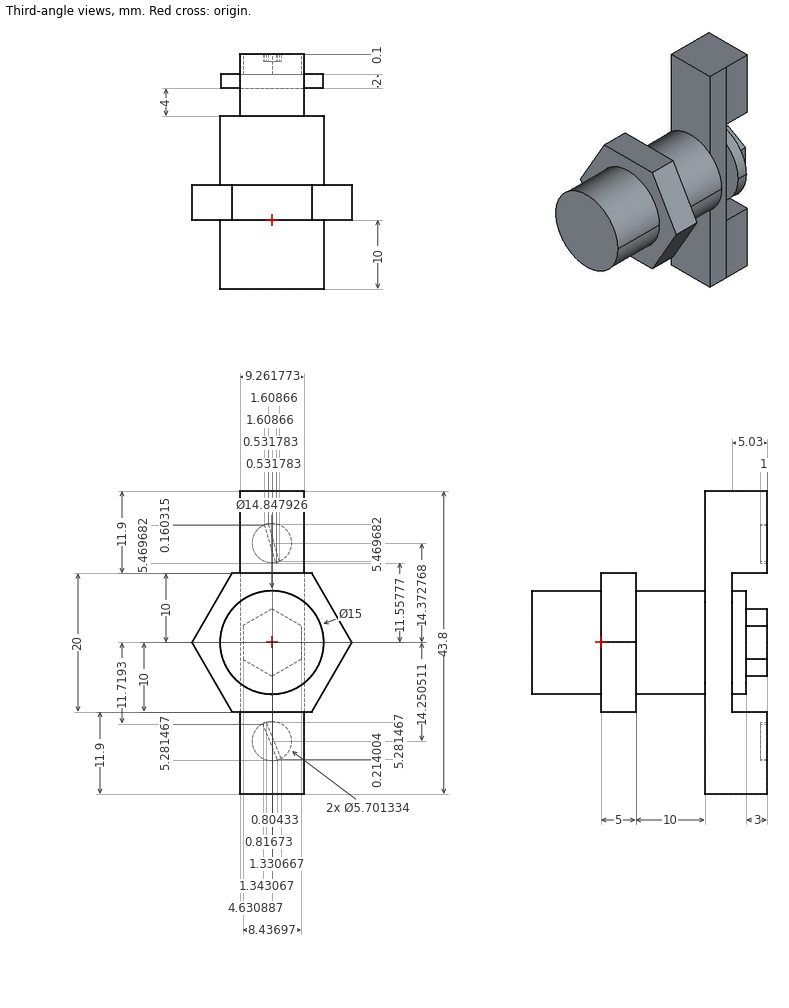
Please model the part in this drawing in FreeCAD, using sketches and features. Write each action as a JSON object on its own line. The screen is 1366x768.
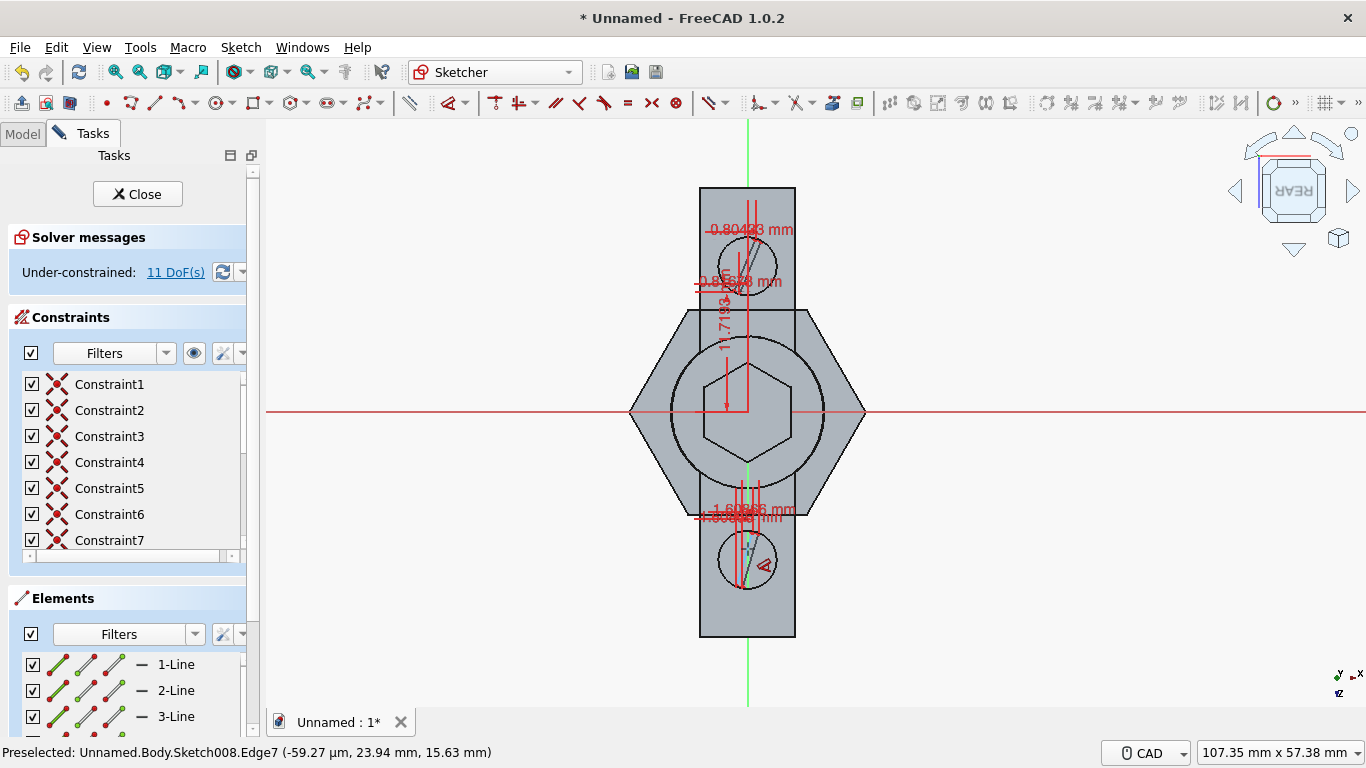
{"action": "scroll", "coordinate": [761, 241], "scroll_direction": "up", "scroll_amount": 6}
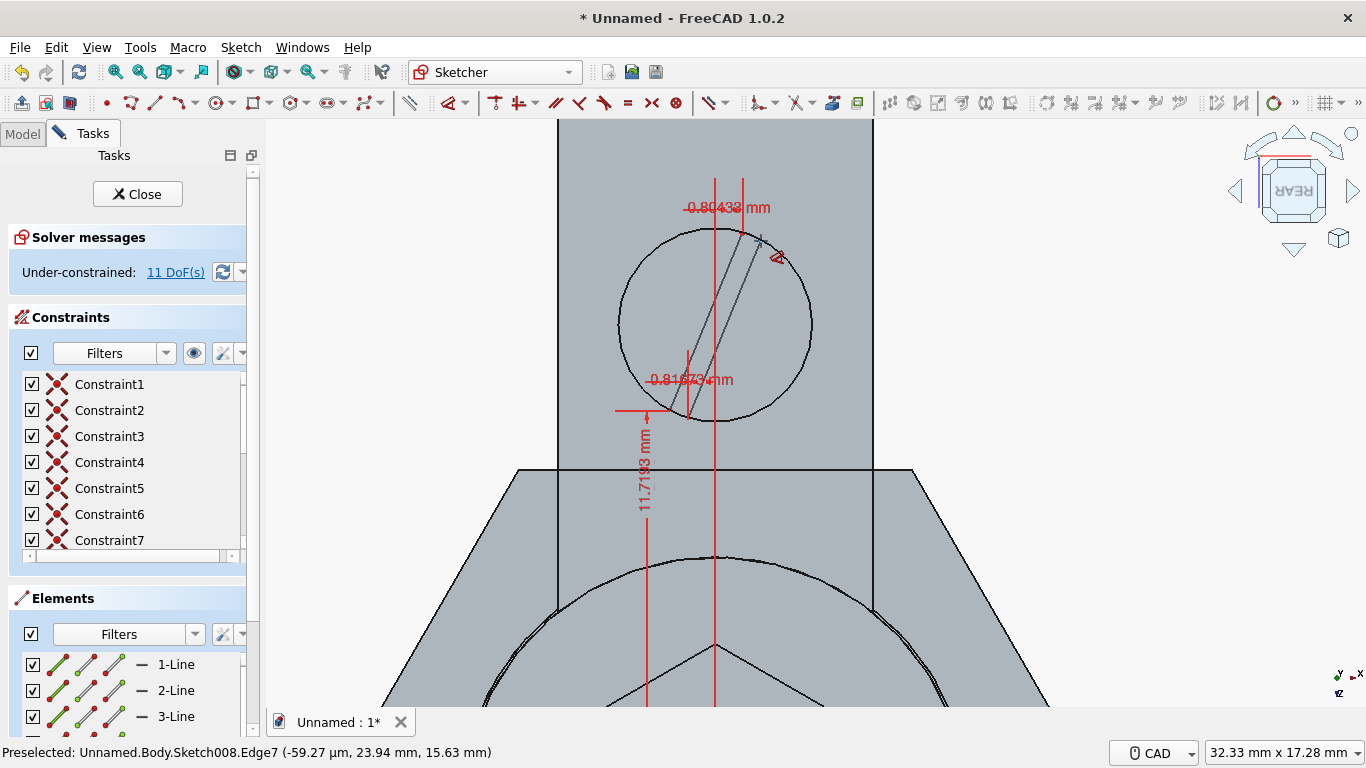
{"action": "left_click", "coordinate": [761, 239]}
{"action": "left_click", "coordinate": [738, 181]}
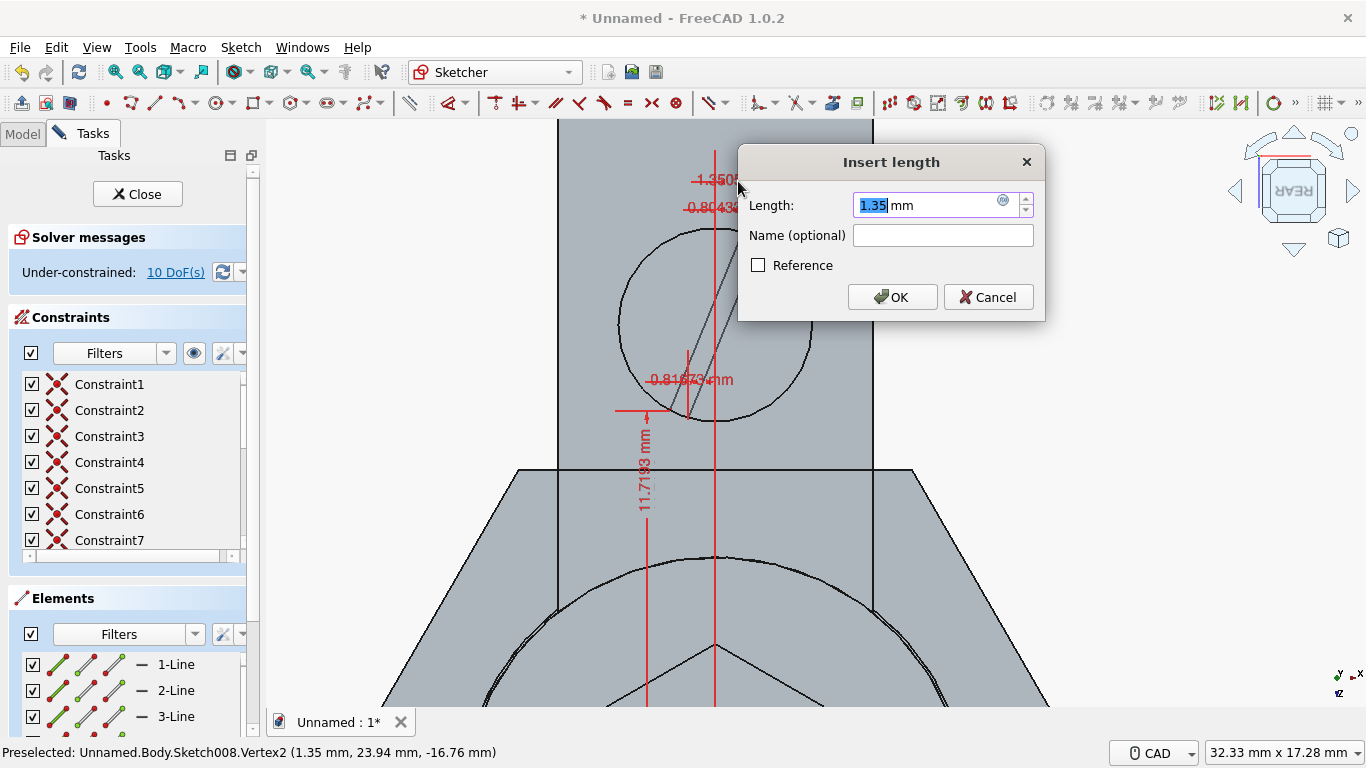
{"action": "type", "text": "1.330667"}
{"action": "key", "text": "Return"}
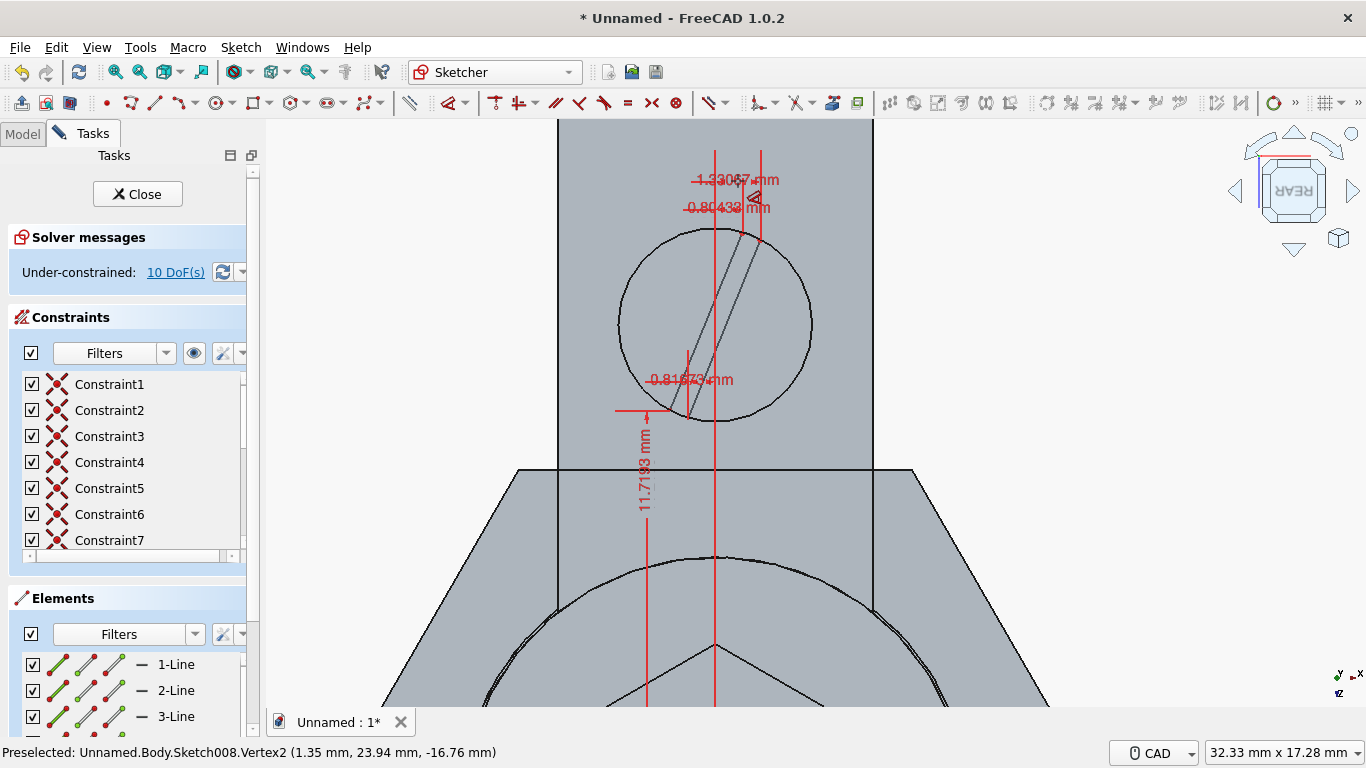
{"action": "left_click", "coordinate": [670, 411]}
{"action": "left_click", "coordinate": [676, 353]}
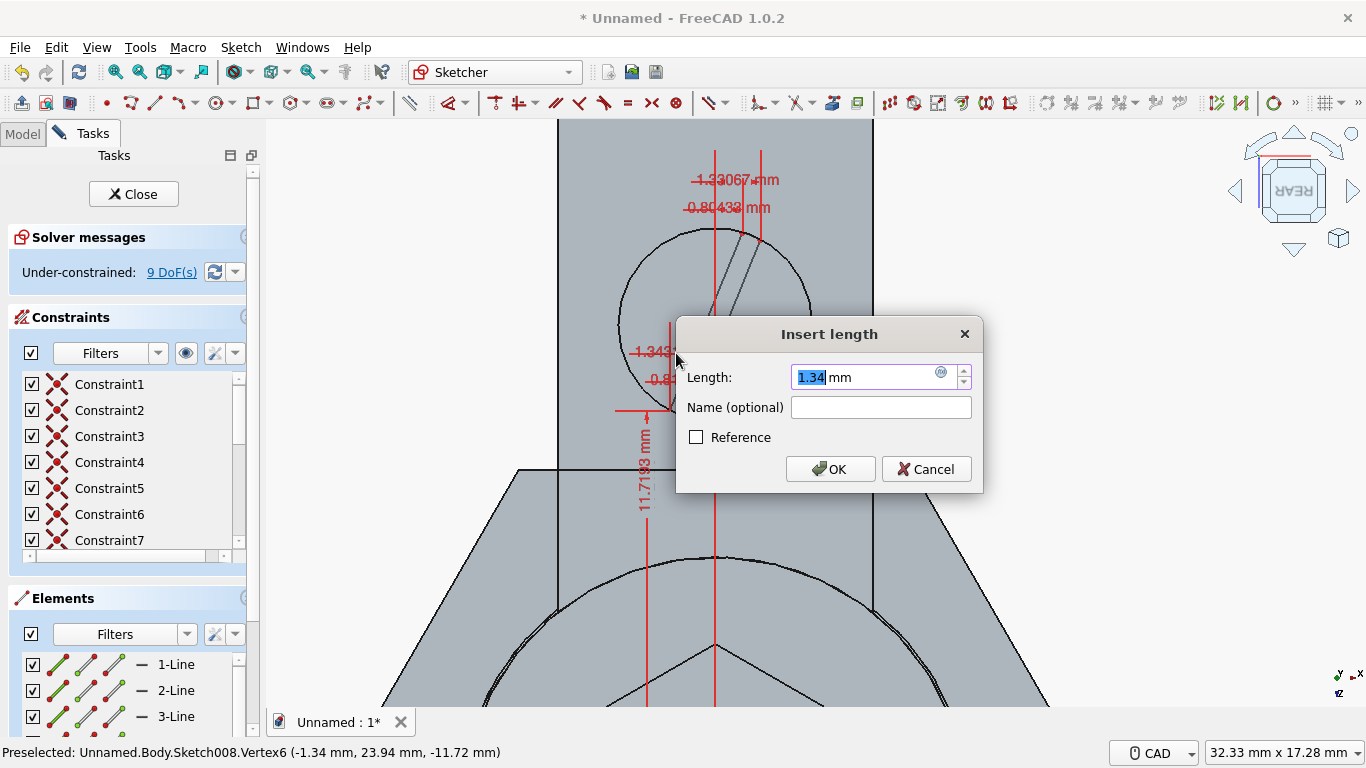
{"action": "type", "text": "1.343067"}
{"action": "key", "text": "Return"}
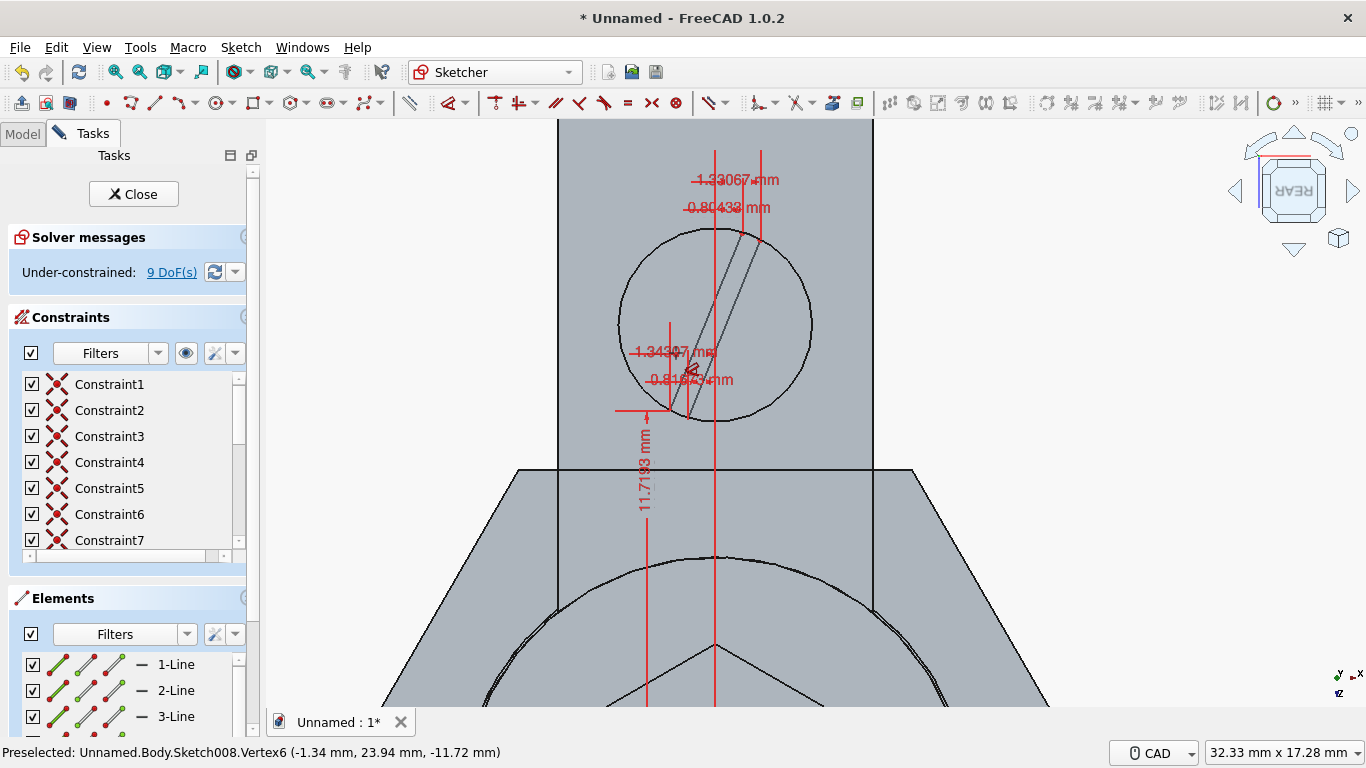
{"action": "scroll", "coordinate": [761, 241], "scroll_direction": "down", "scroll_amount": 6}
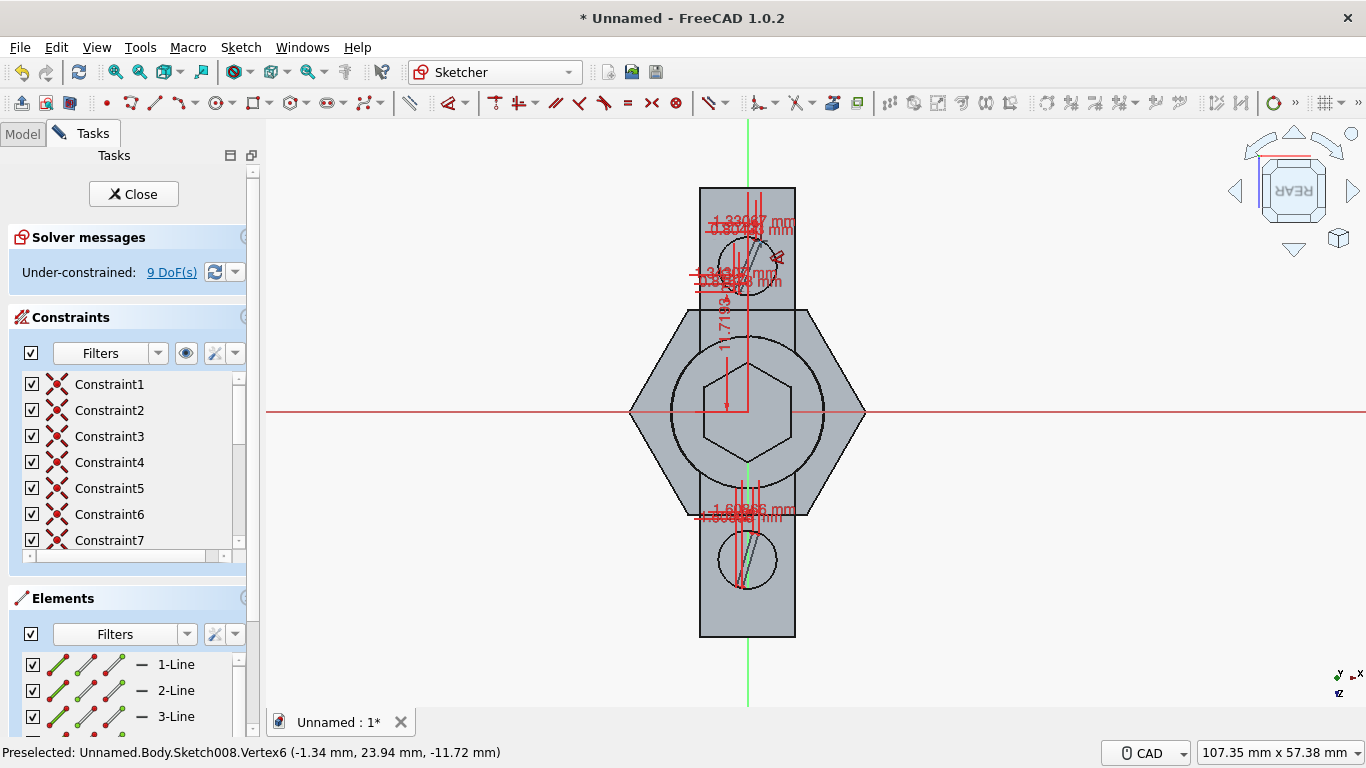
{"action": "scroll", "coordinate": [753, 531], "scroll_direction": "up", "scroll_amount": 10}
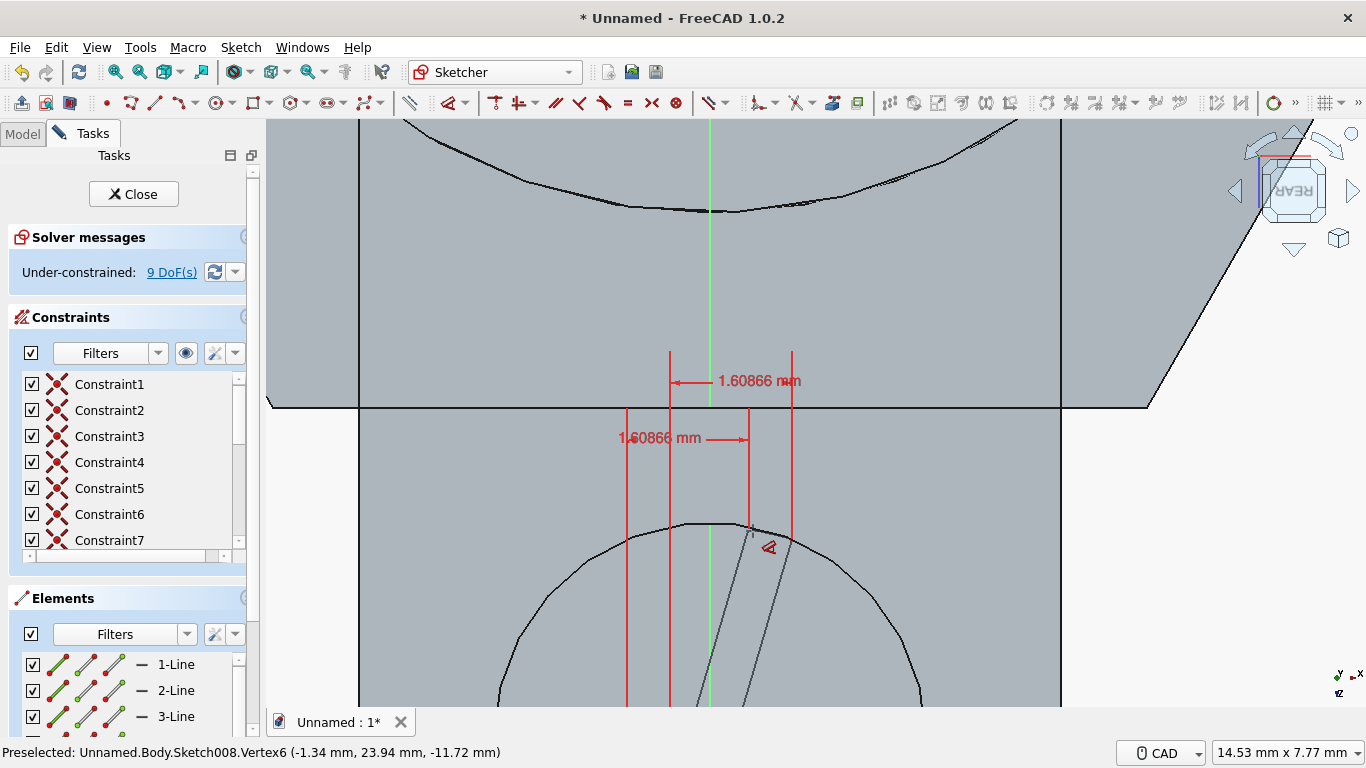
{"action": "left_click", "coordinate": [749, 529]}
{"action": "left_click", "coordinate": [743, 611]}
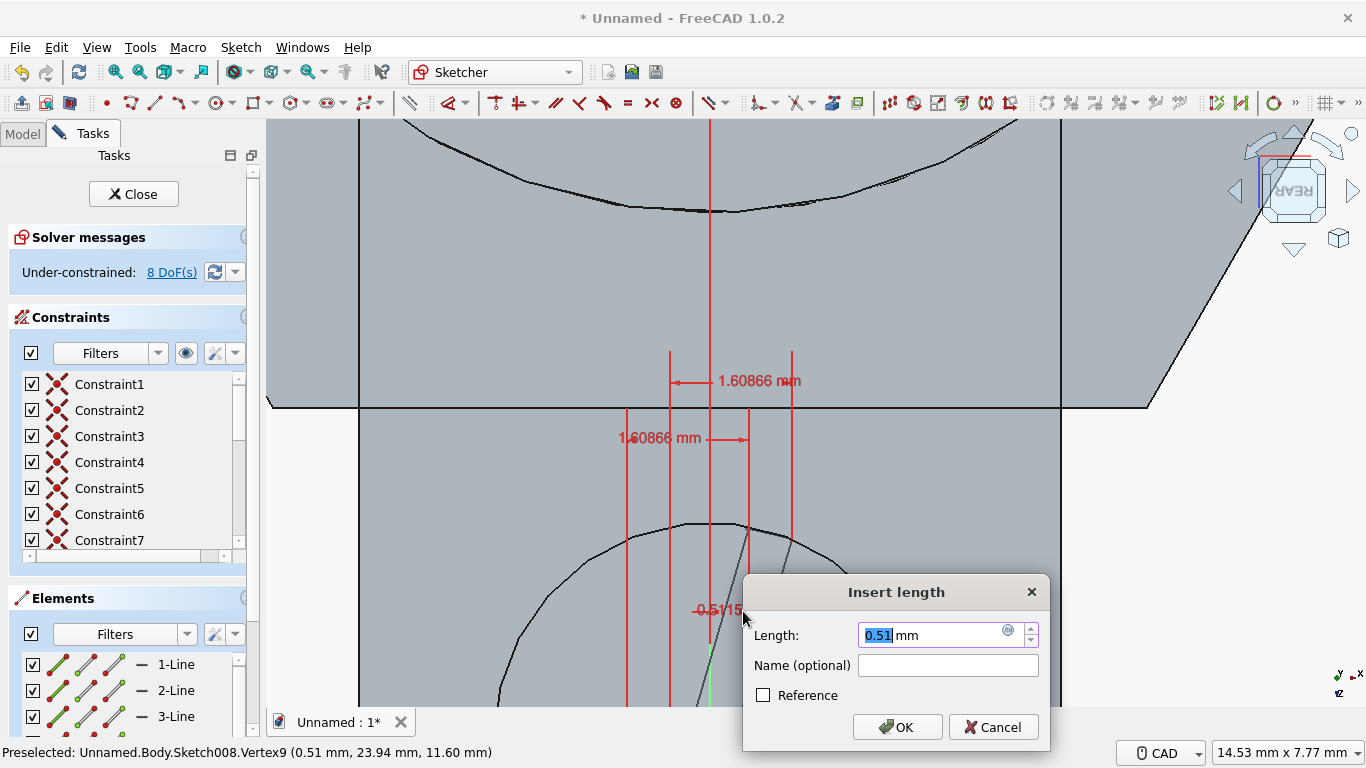
{"action": "type", "text": "0.531783"}
{"action": "key", "text": "Return"}